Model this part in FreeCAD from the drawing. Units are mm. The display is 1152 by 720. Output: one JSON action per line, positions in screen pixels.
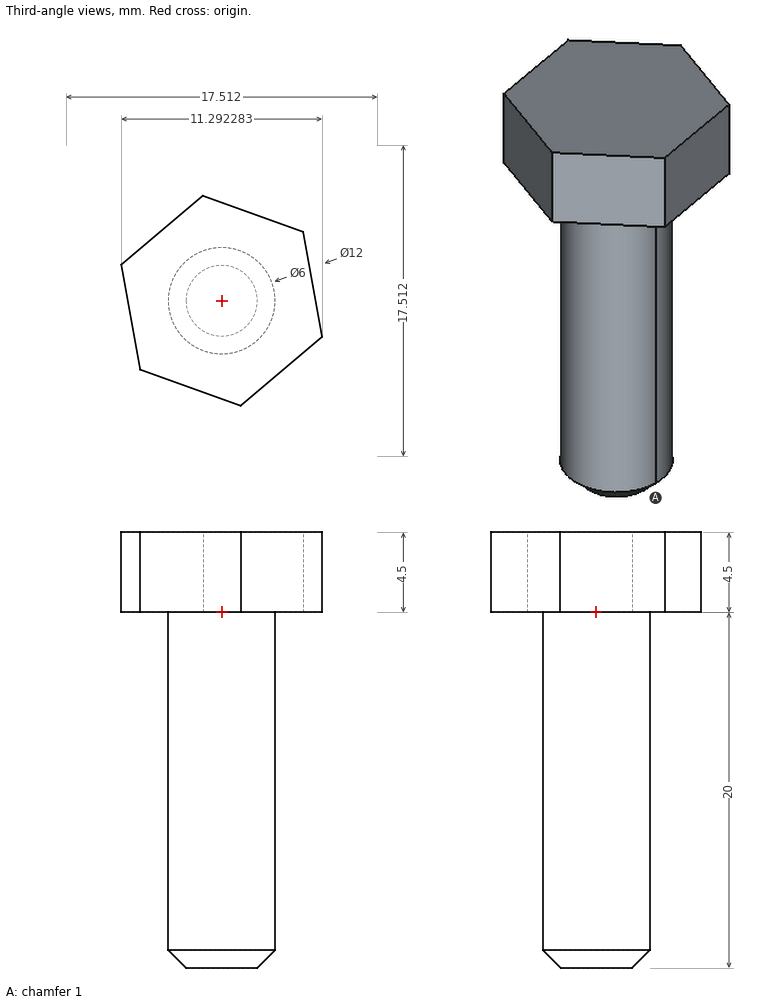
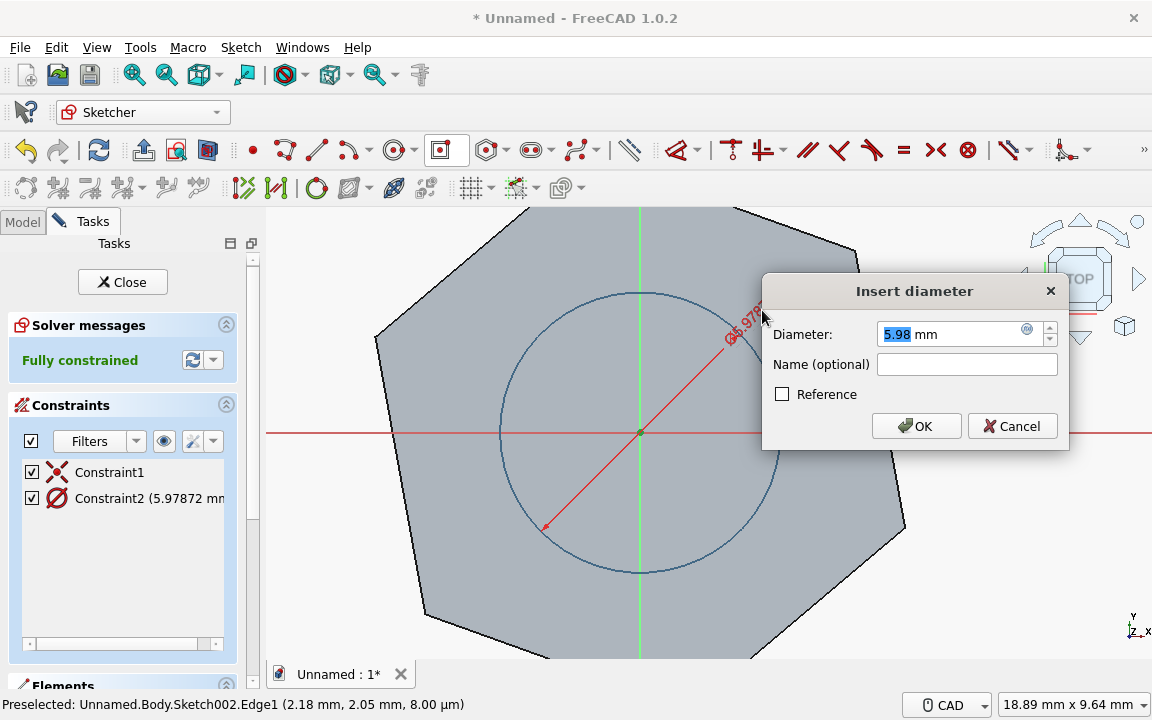
{"action": "type", "text": "6"}
{"action": "key", "text": "Return"}
{"action": "key", "text": "Escape"}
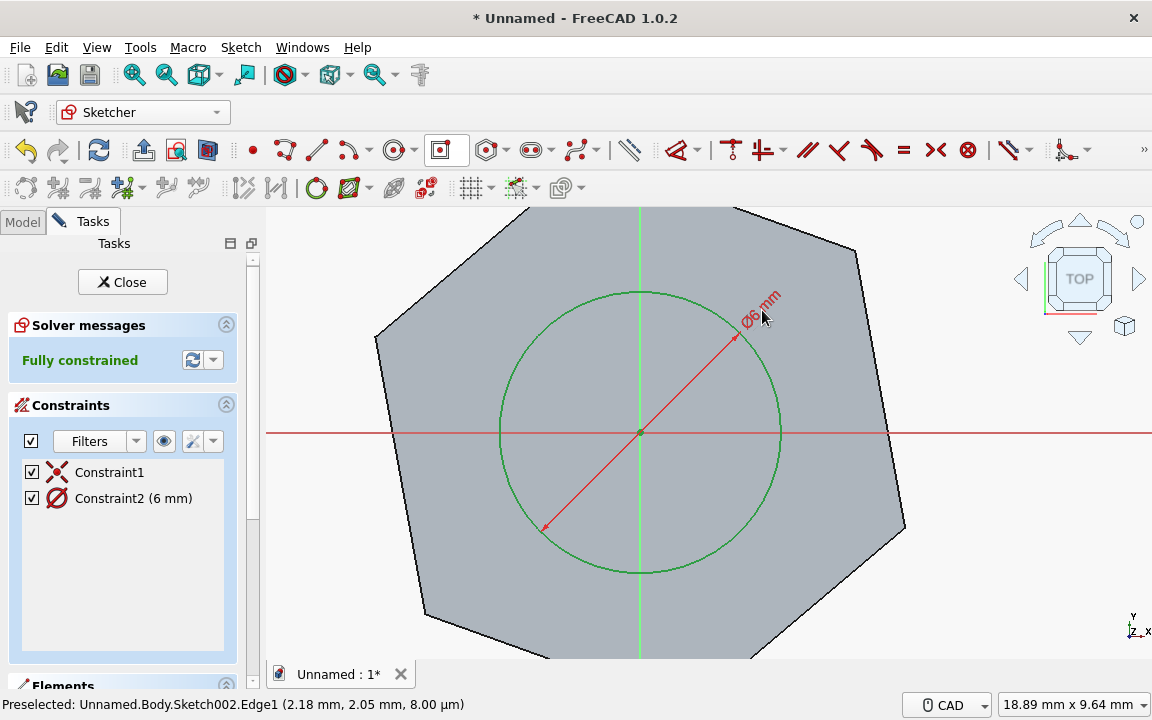
{"action": "left_click", "coordinate": [123, 282]}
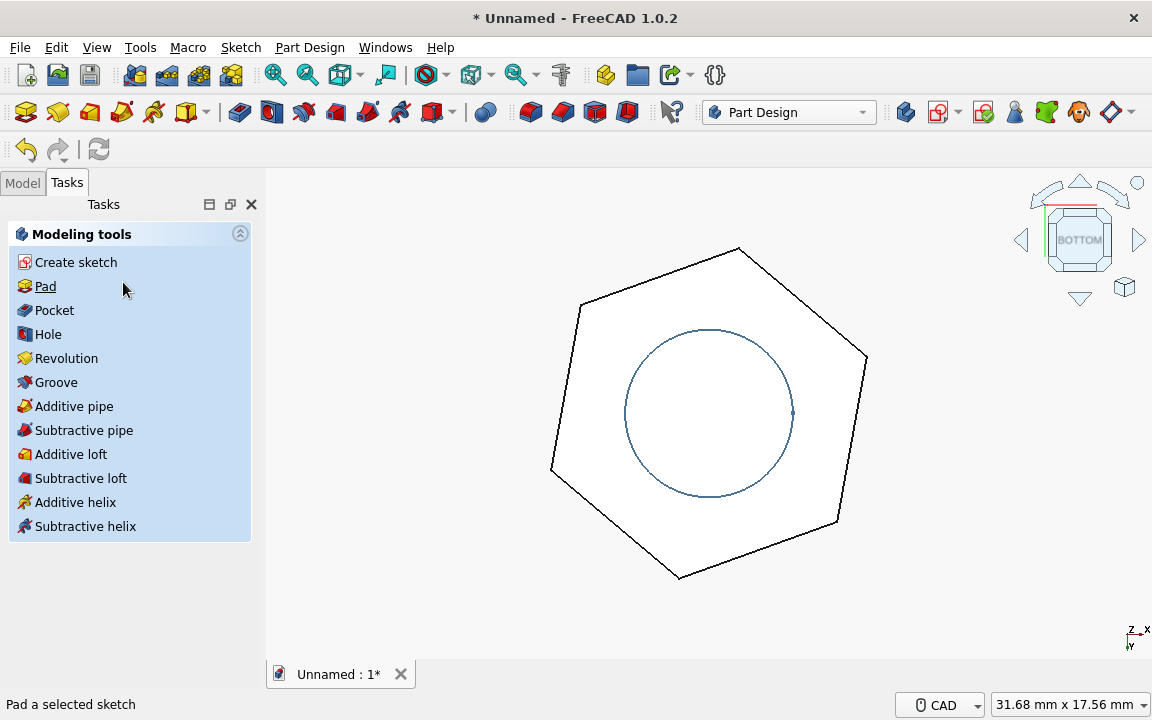
{"action": "left_click", "coordinate": [26, 112]}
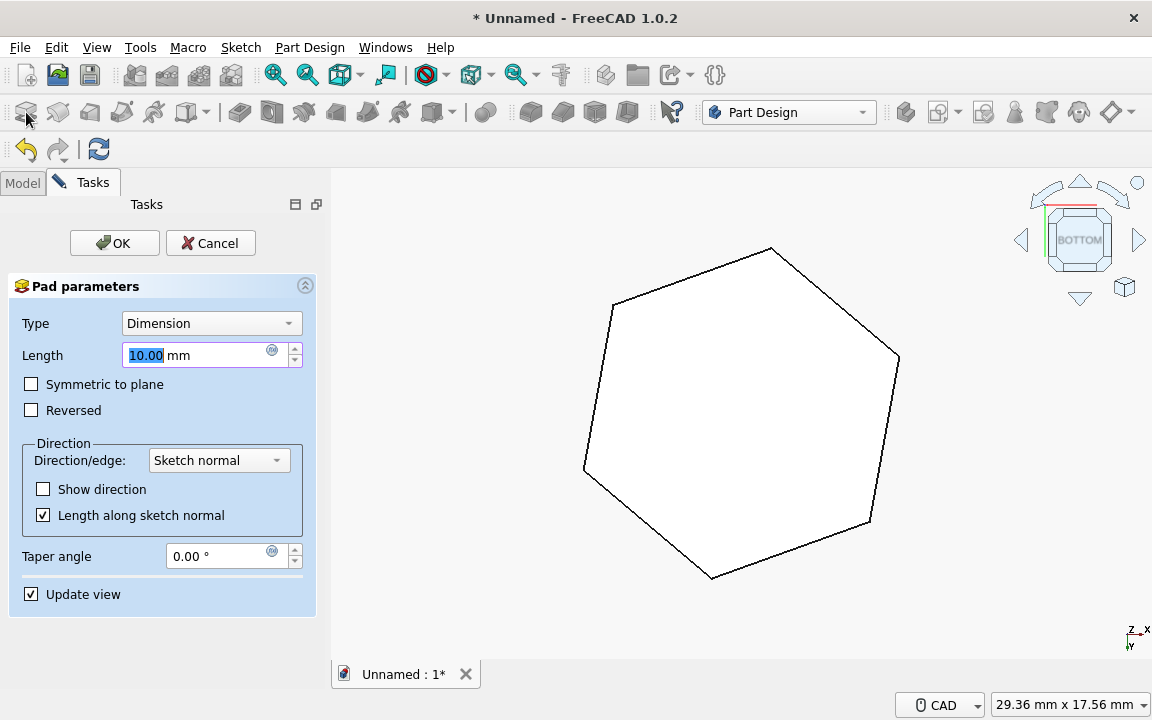
{"action": "type", "text": "20"}
{"action": "key", "text": "Tab"}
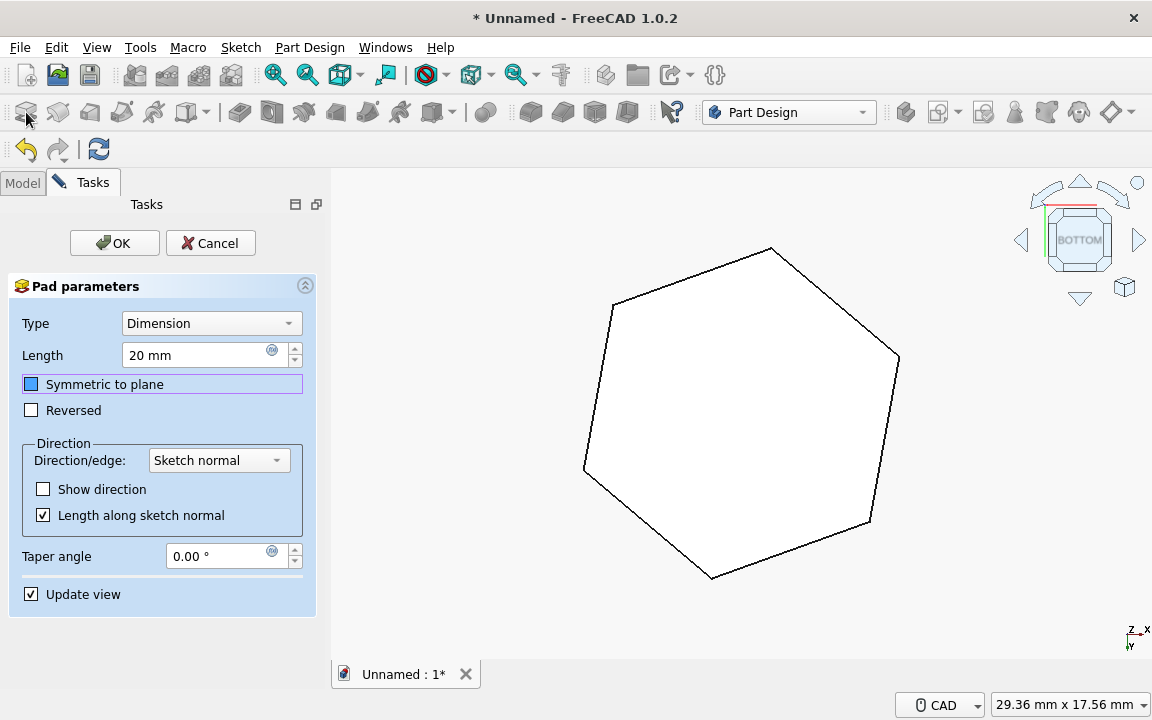
{"action": "left_click", "coordinate": [30, 410]}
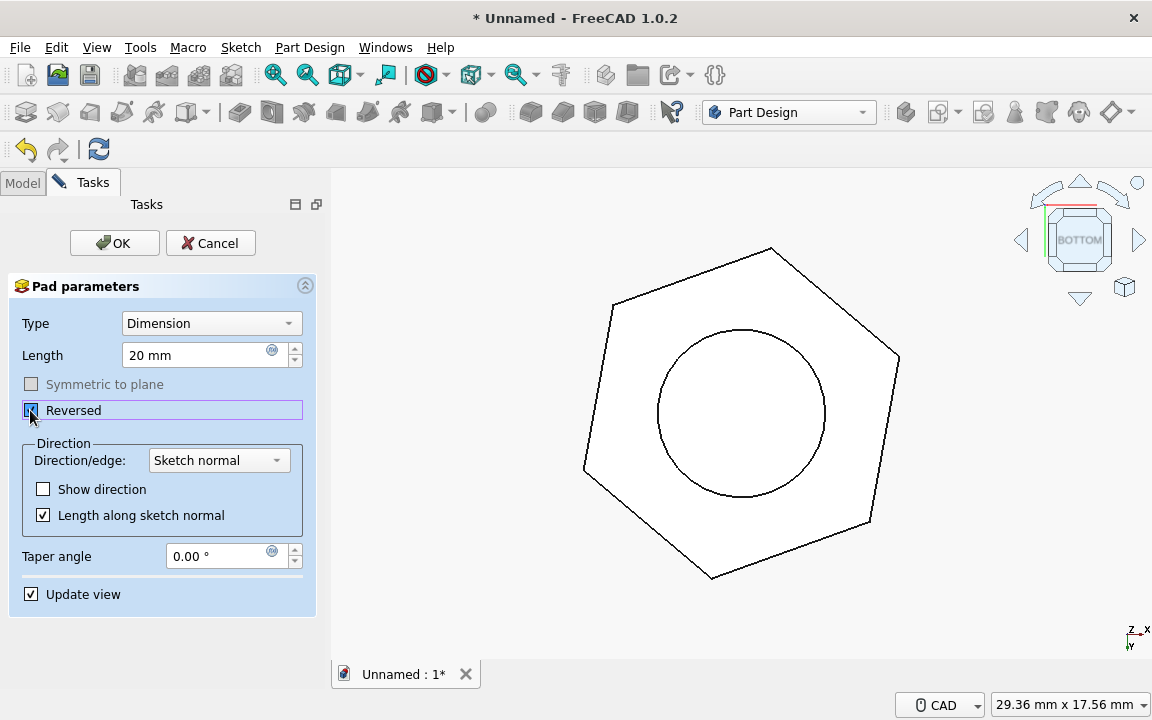
{"action": "left_click", "coordinate": [115, 243]}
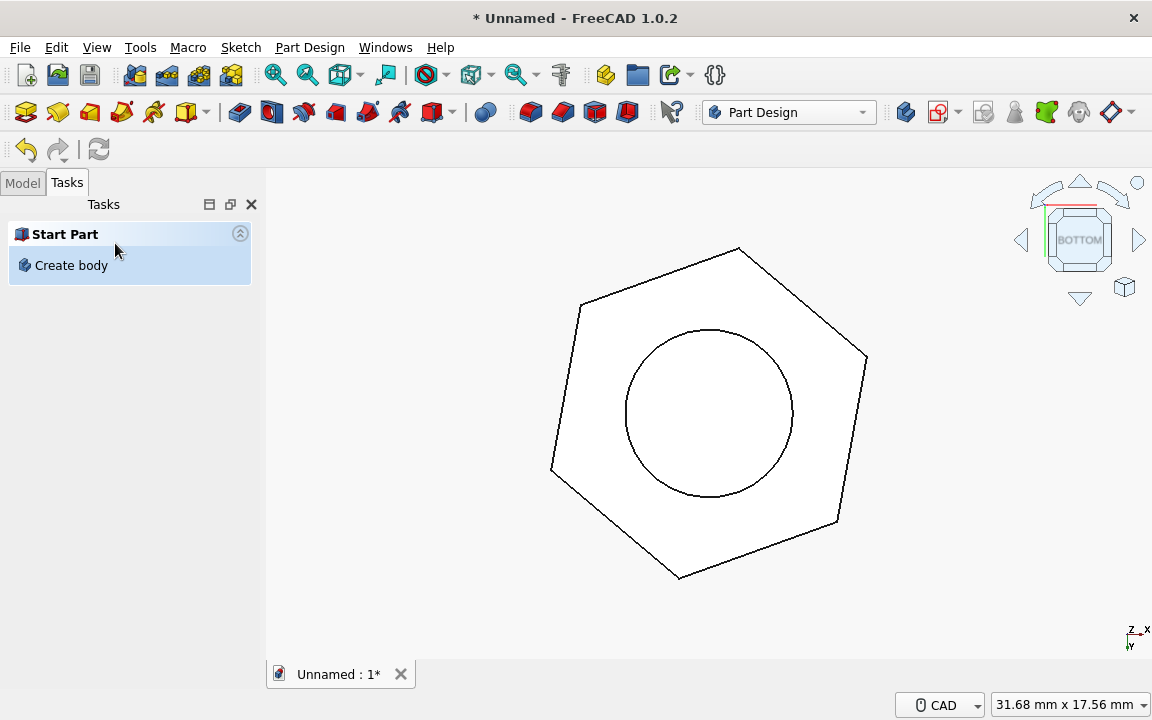
{"action": "left_click", "coordinate": [625, 412]}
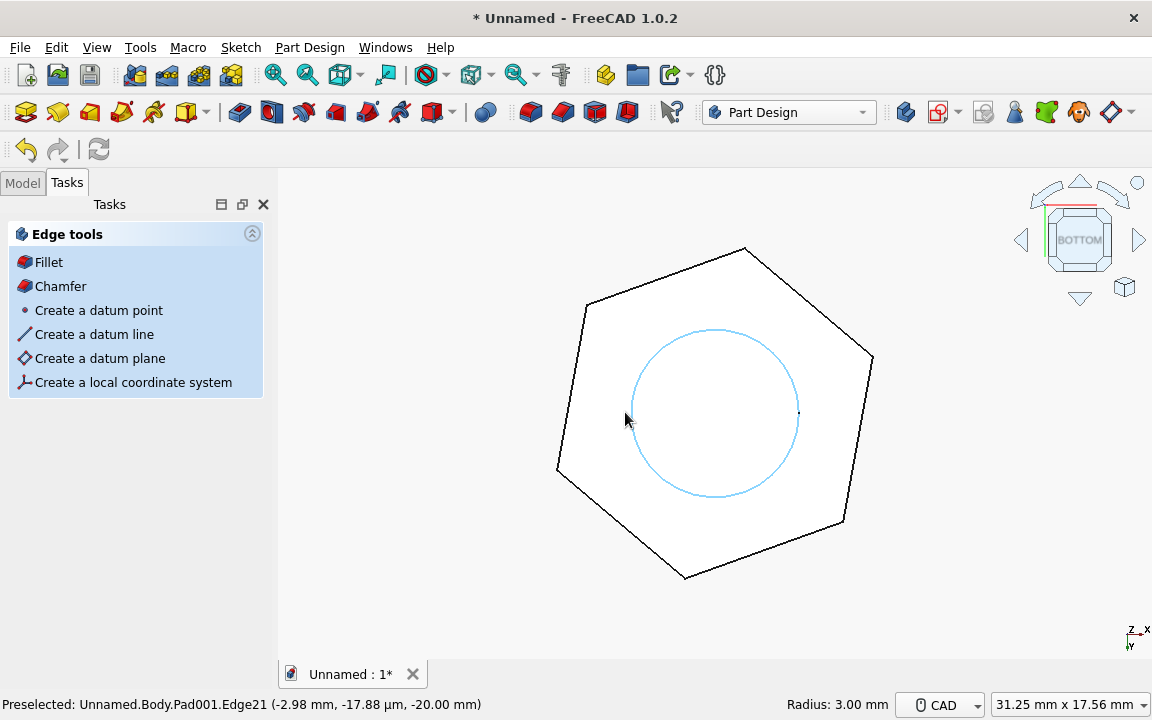
{"action": "left_click", "coordinate": [564, 112]}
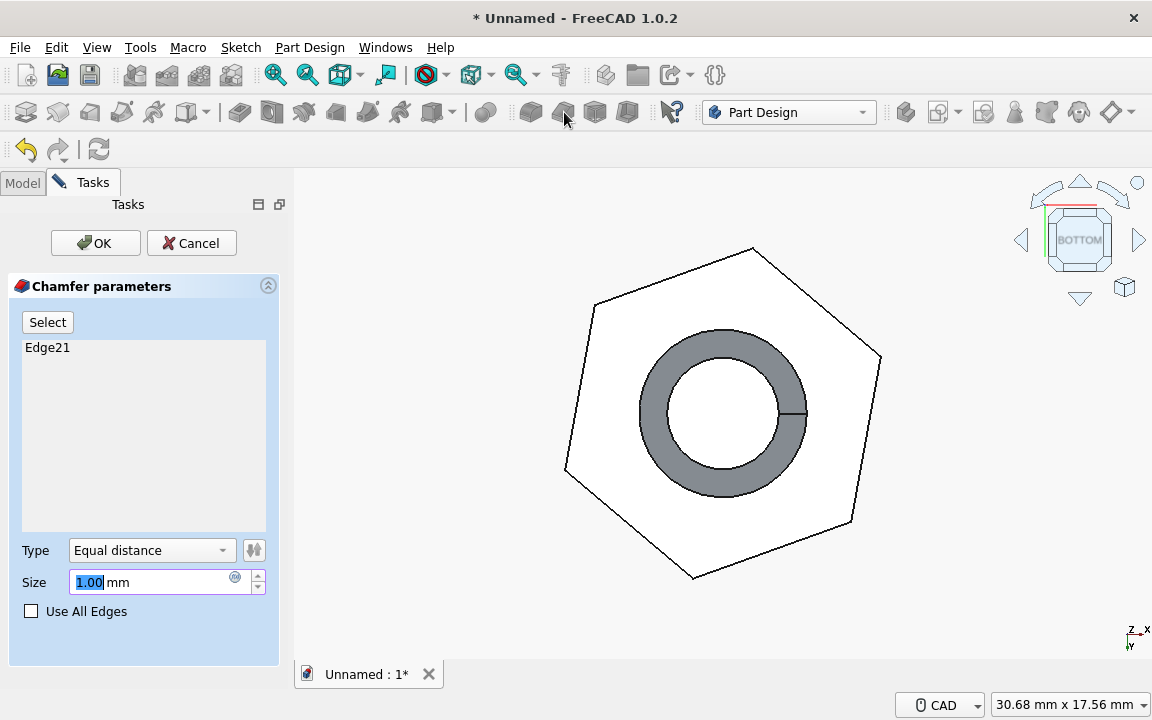
{"action": "type", "text": "1"}
{"action": "key", "text": "Tab"}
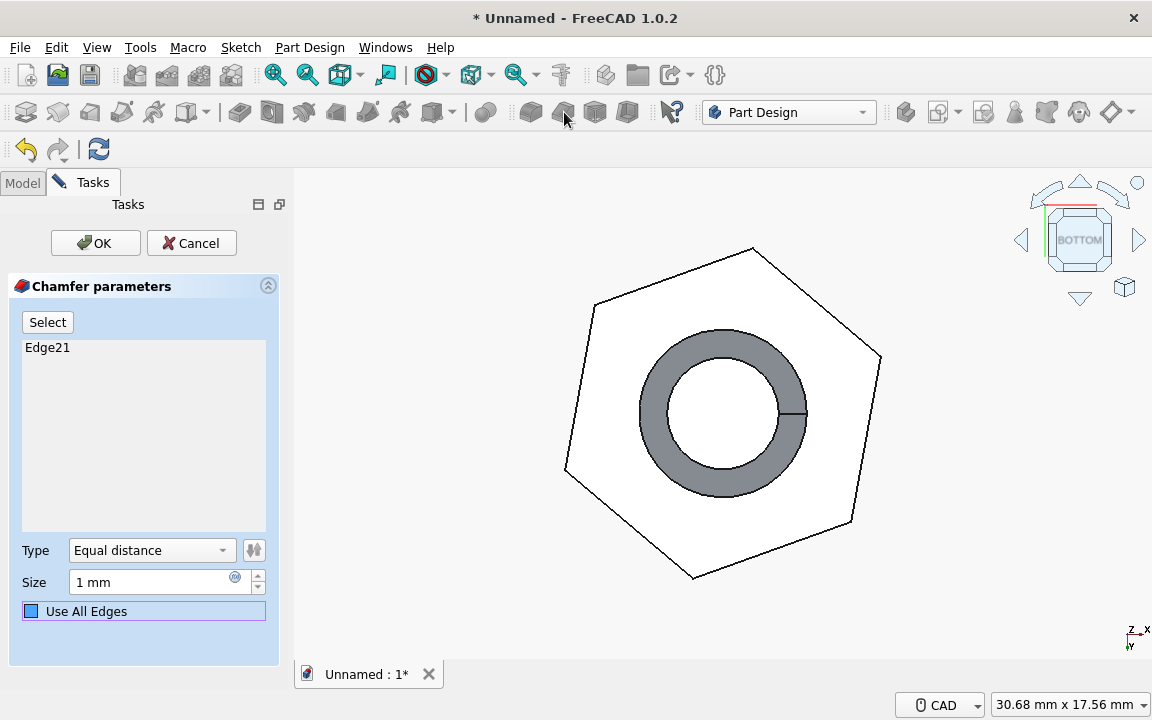
{"action": "left_click", "coordinate": [96, 243]}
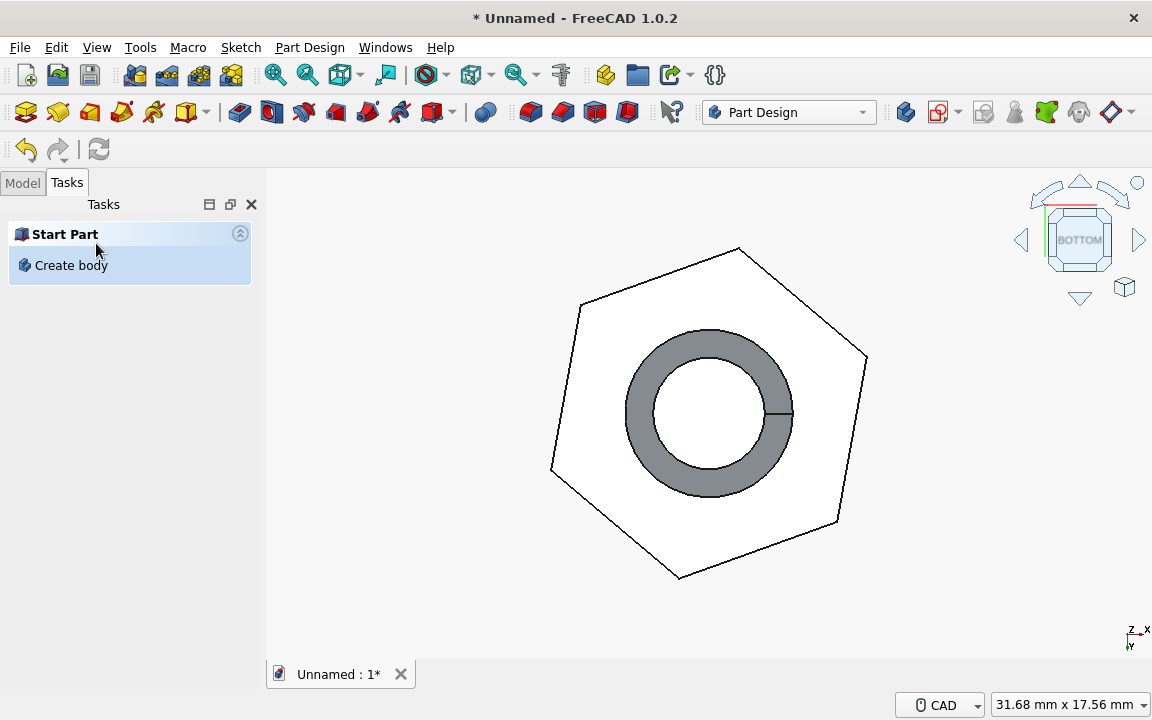
{"action": "key", "text": "0"}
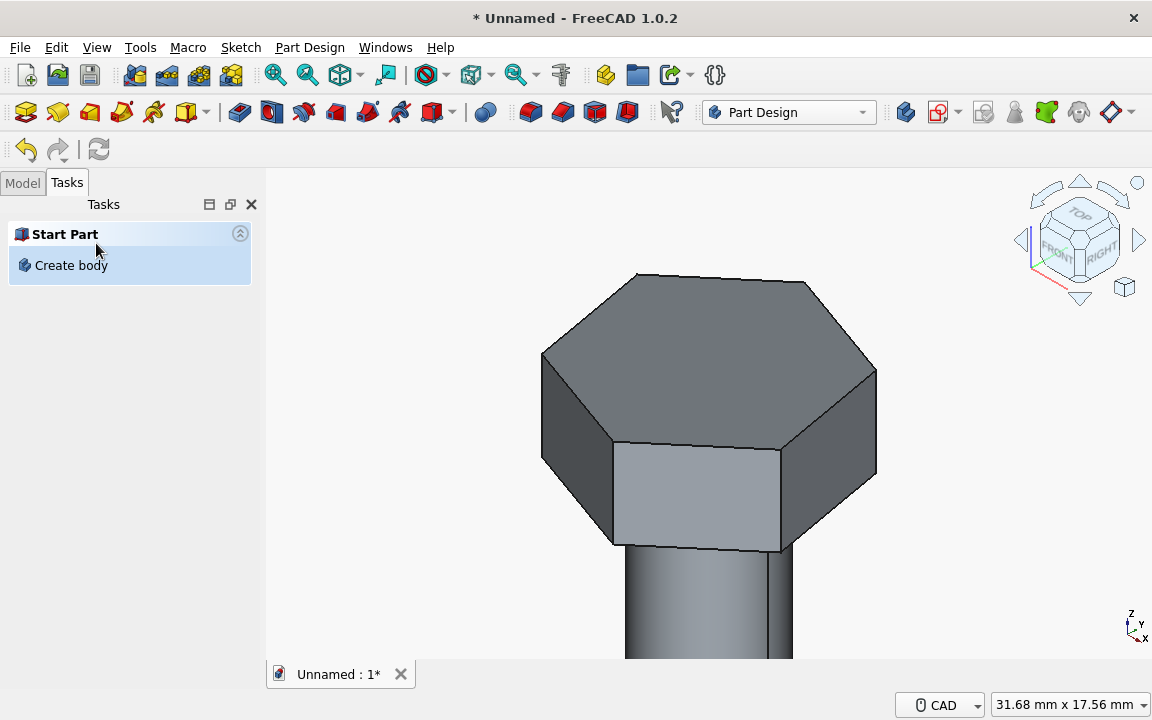
{"action": "left_click", "coordinate": [276, 76]}